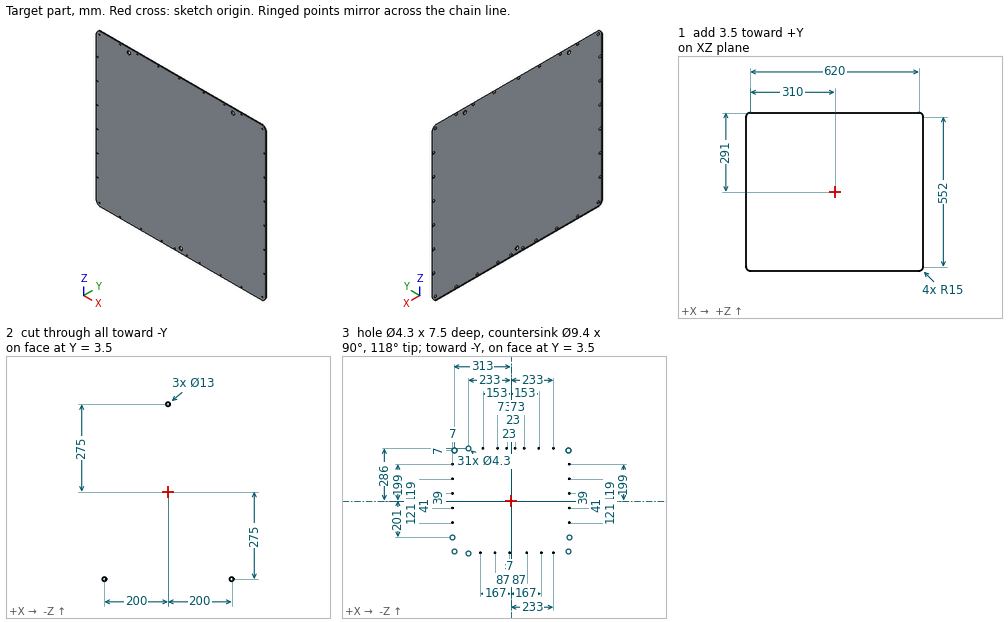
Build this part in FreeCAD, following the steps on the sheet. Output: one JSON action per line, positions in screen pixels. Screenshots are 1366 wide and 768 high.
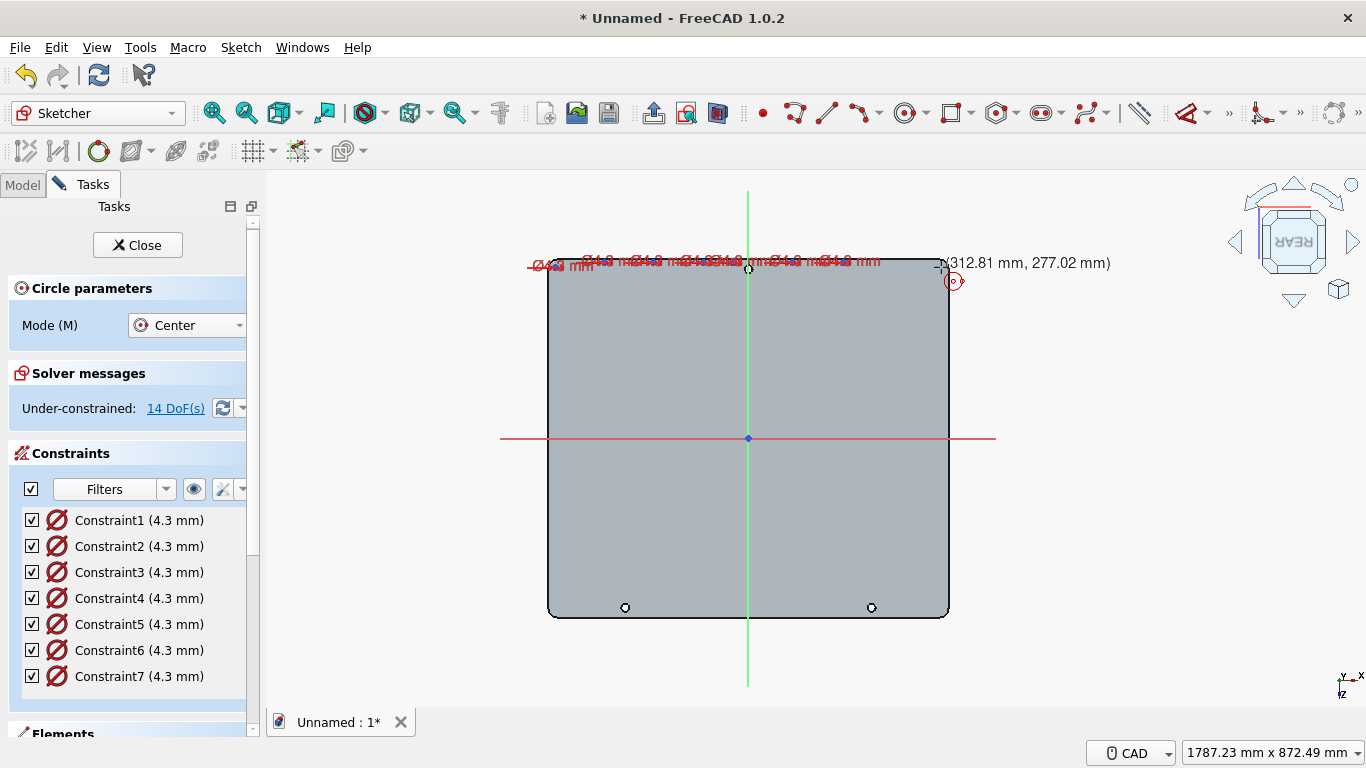
{"action": "left_click", "coordinate": [941, 267]}
{"action": "mouse_move", "coordinate": [942, 266]}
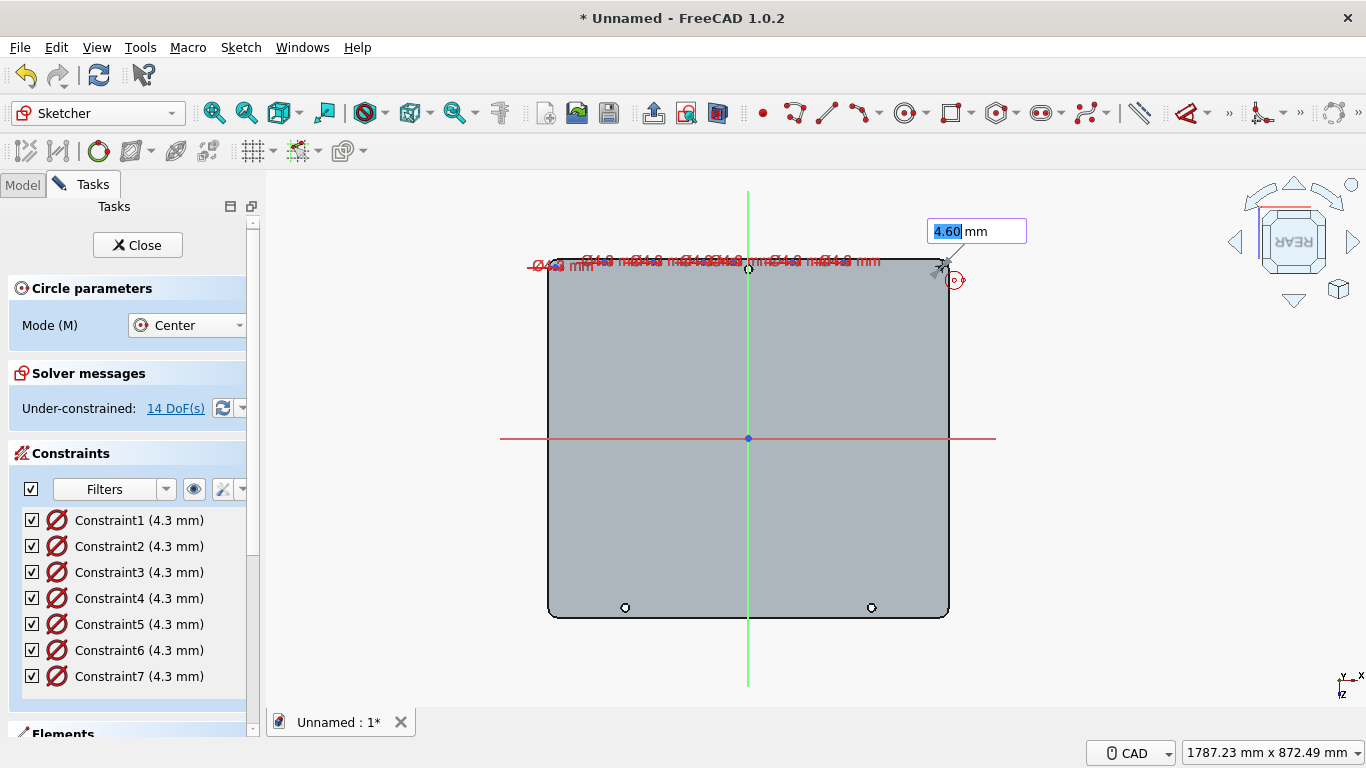
{"action": "type", "text": "4.3"}
{"action": "key", "text": "Return"}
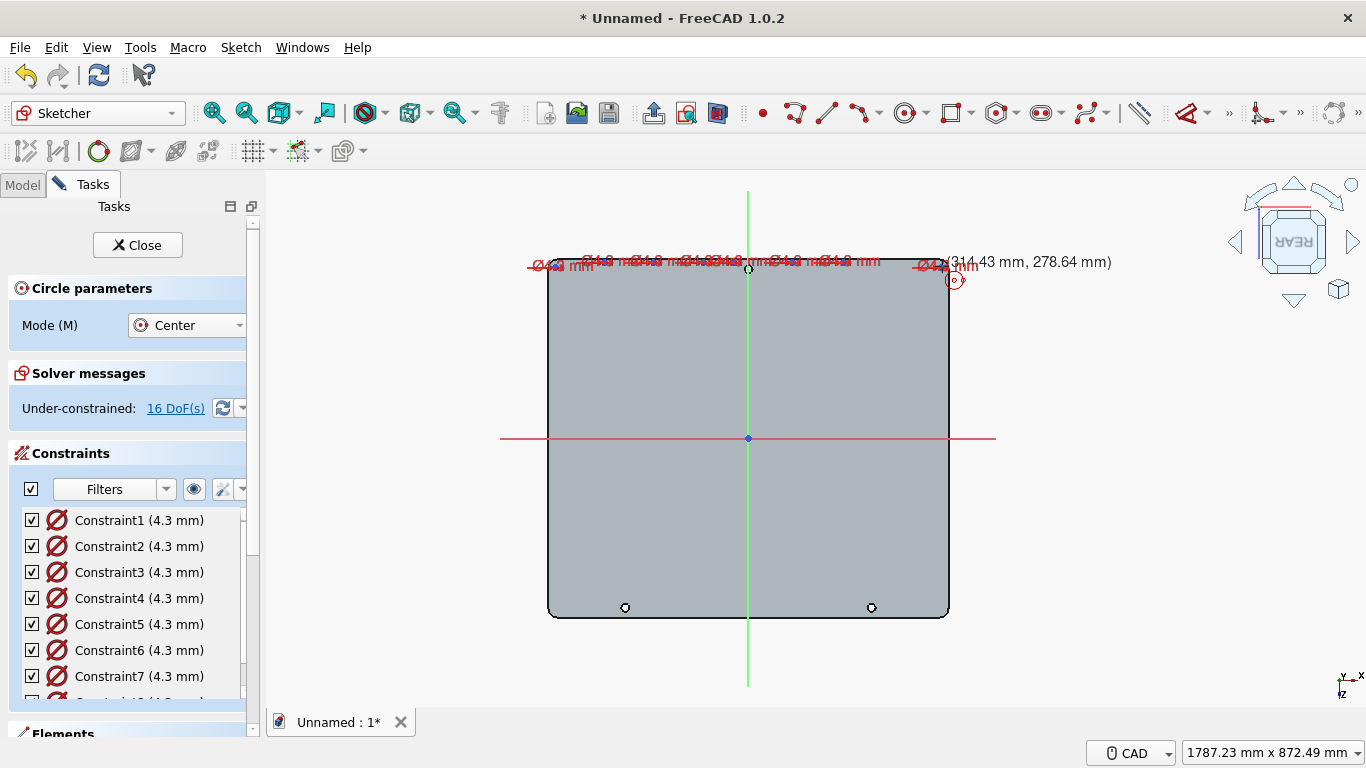
{"action": "scroll", "coordinate": [552, 316], "scroll_direction": "up", "scroll_amount": 15}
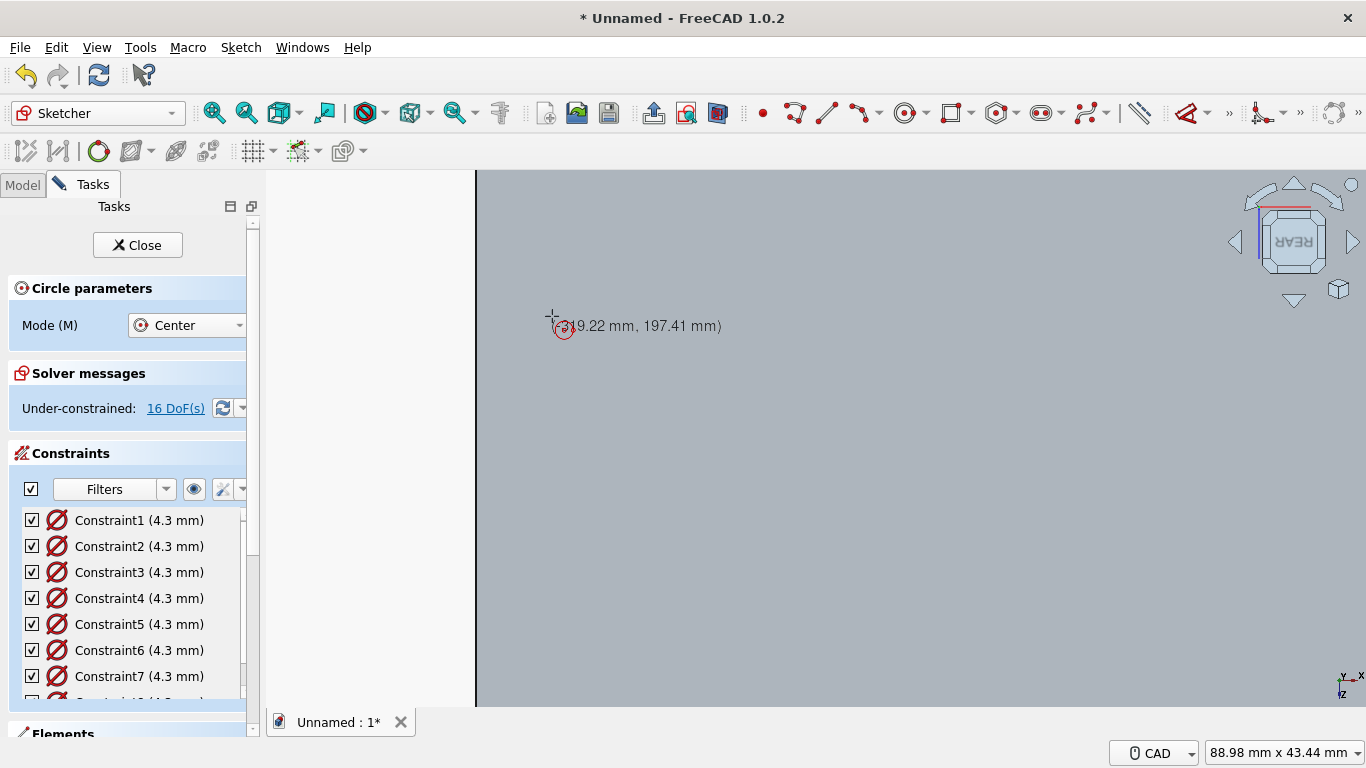
{"action": "scroll", "coordinate": [551, 316], "scroll_direction": "down", "scroll_amount": 15}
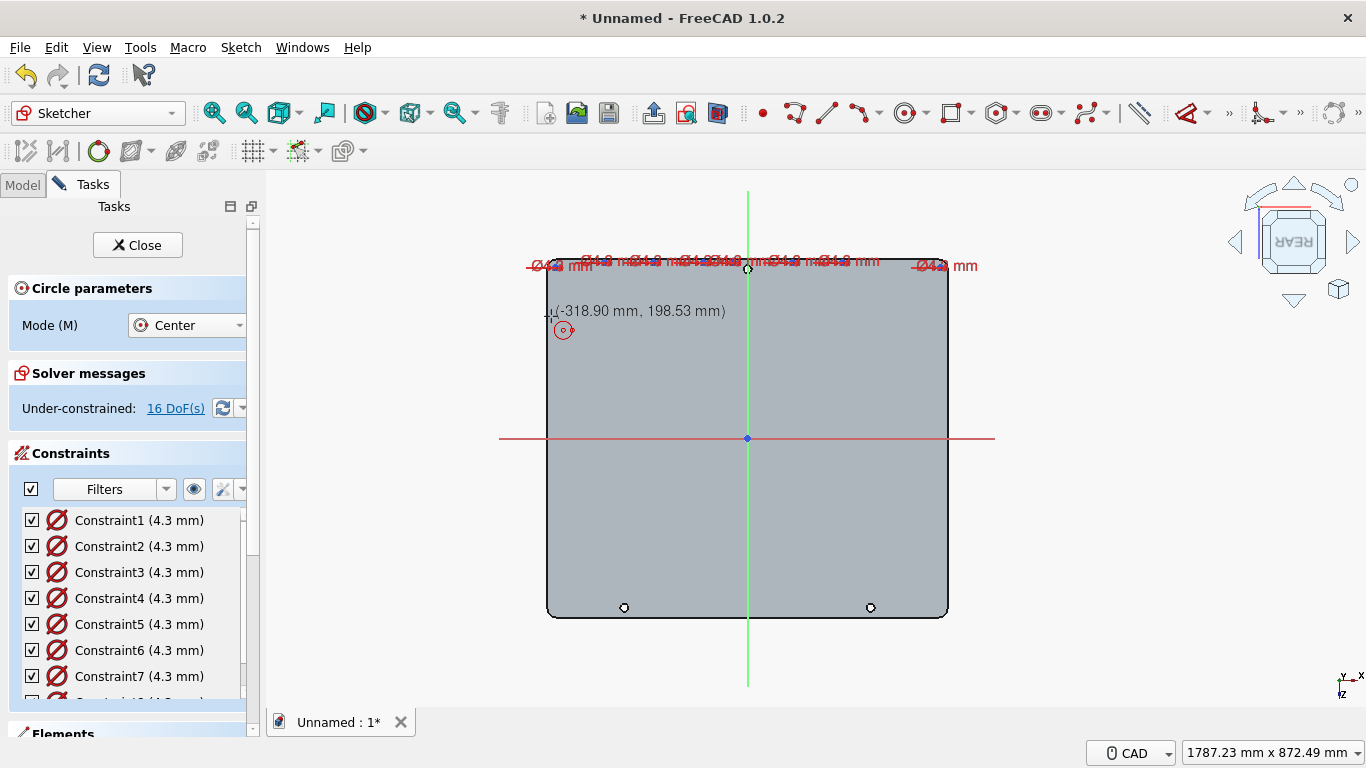
{"action": "left_click", "coordinate": [551, 316]}
{"action": "mouse_move", "coordinate": [552, 315]}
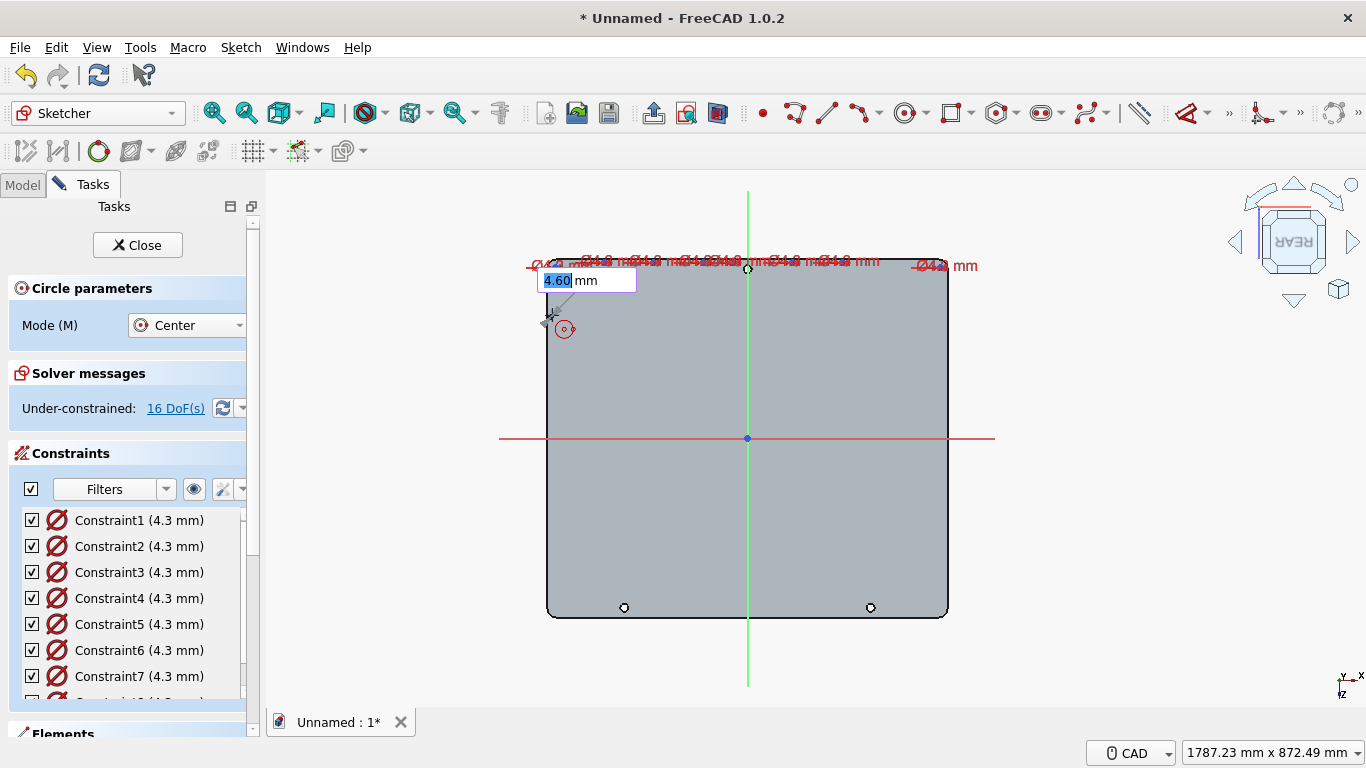
{"action": "type", "text": "4.3"}
{"action": "key", "text": "Return"}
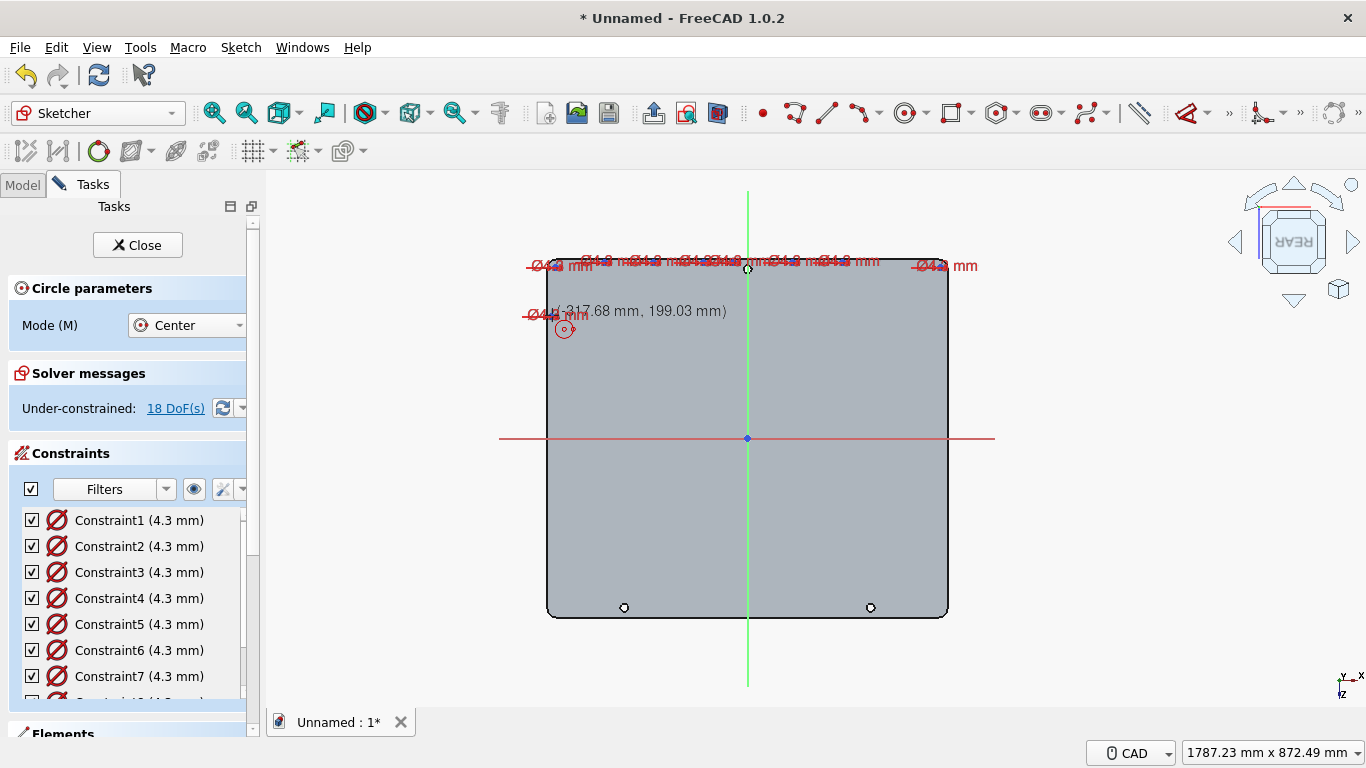
{"action": "scroll", "coordinate": [551, 365], "scroll_direction": "up", "scroll_amount": 15}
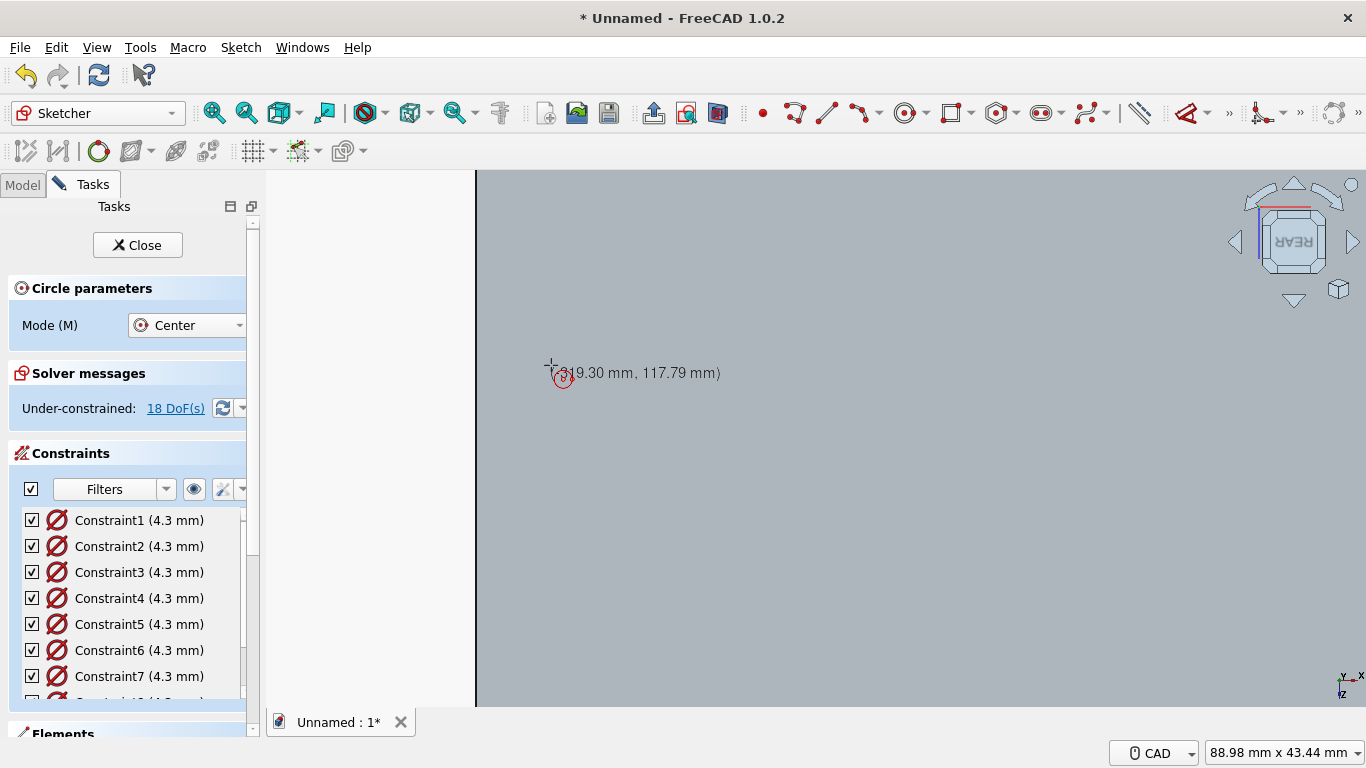
{"action": "scroll", "coordinate": [551, 365], "scroll_direction": "down", "scroll_amount": 15}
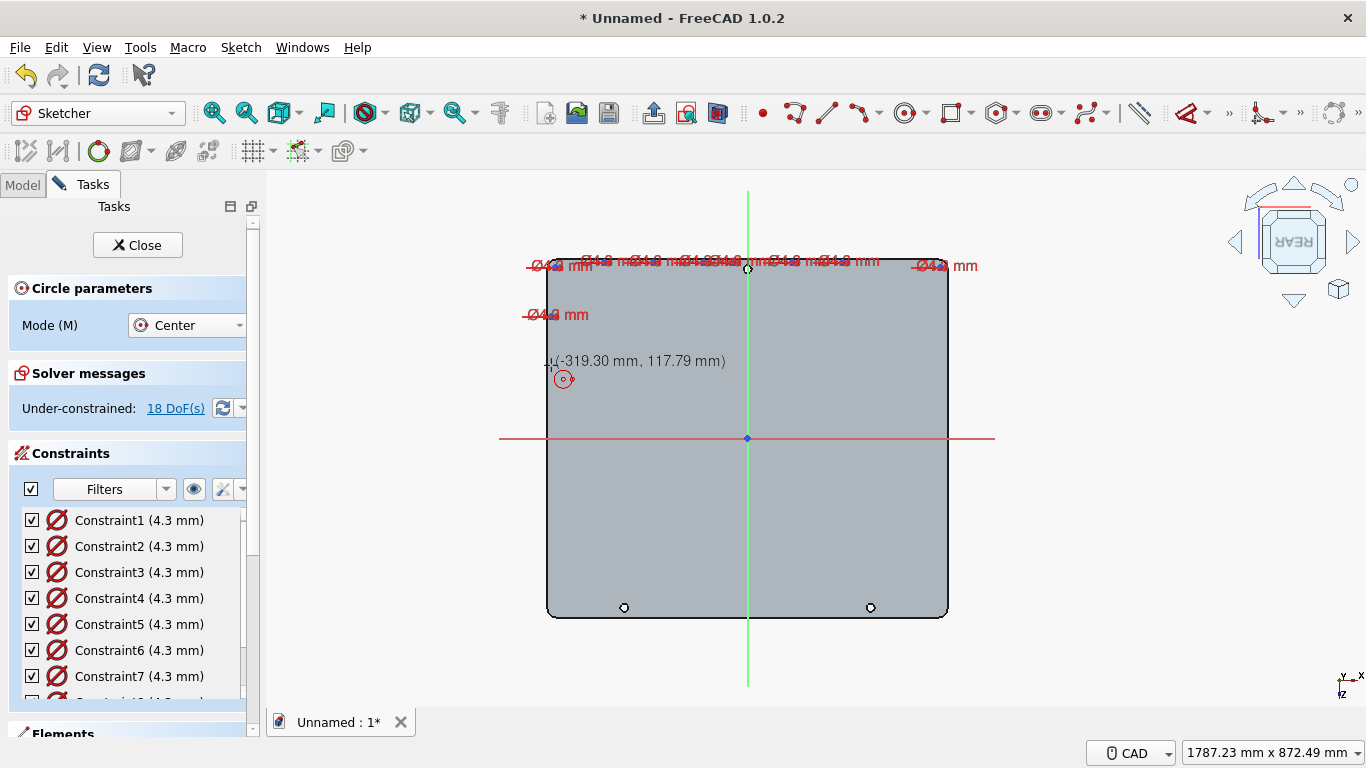
{"action": "left_click", "coordinate": [551, 365]}
{"action": "mouse_move", "coordinate": [552, 364]}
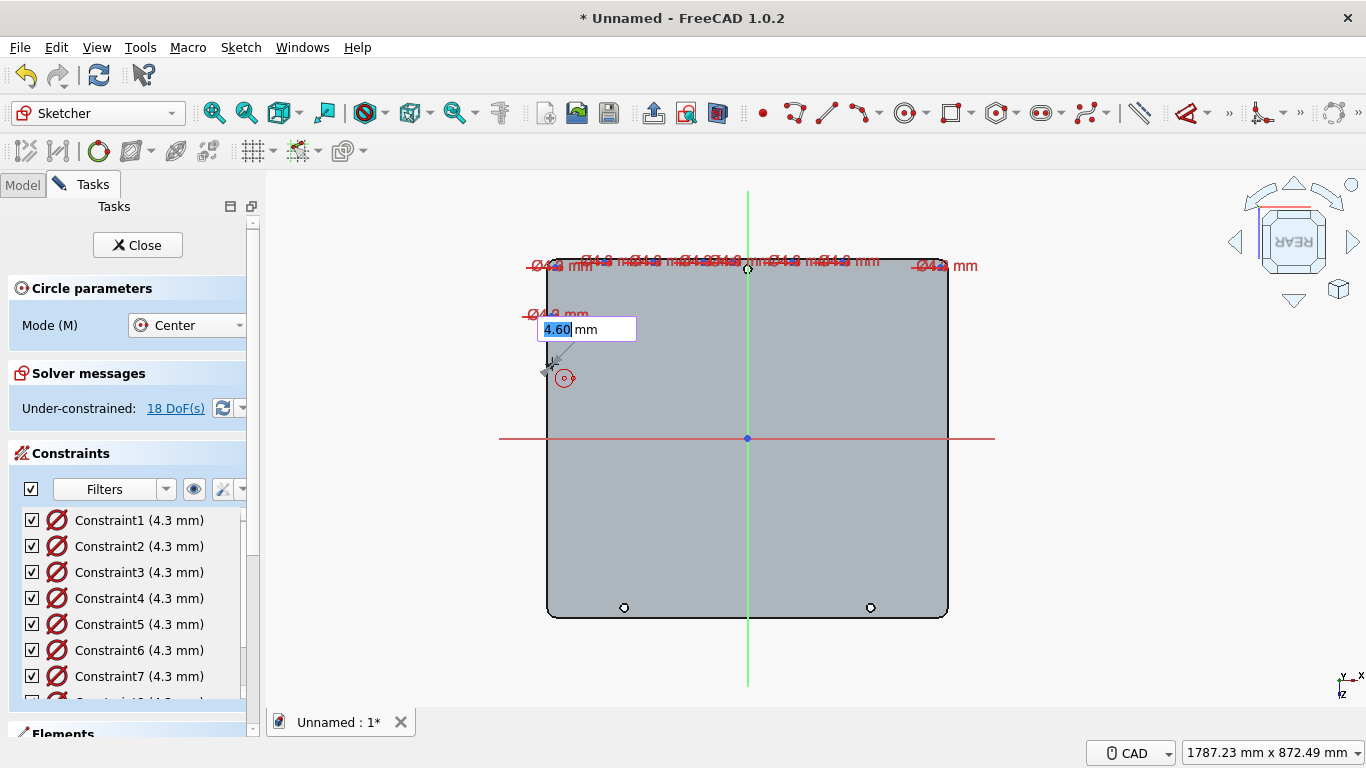
{"action": "type", "text": "4.3"}
{"action": "key", "text": "Return"}